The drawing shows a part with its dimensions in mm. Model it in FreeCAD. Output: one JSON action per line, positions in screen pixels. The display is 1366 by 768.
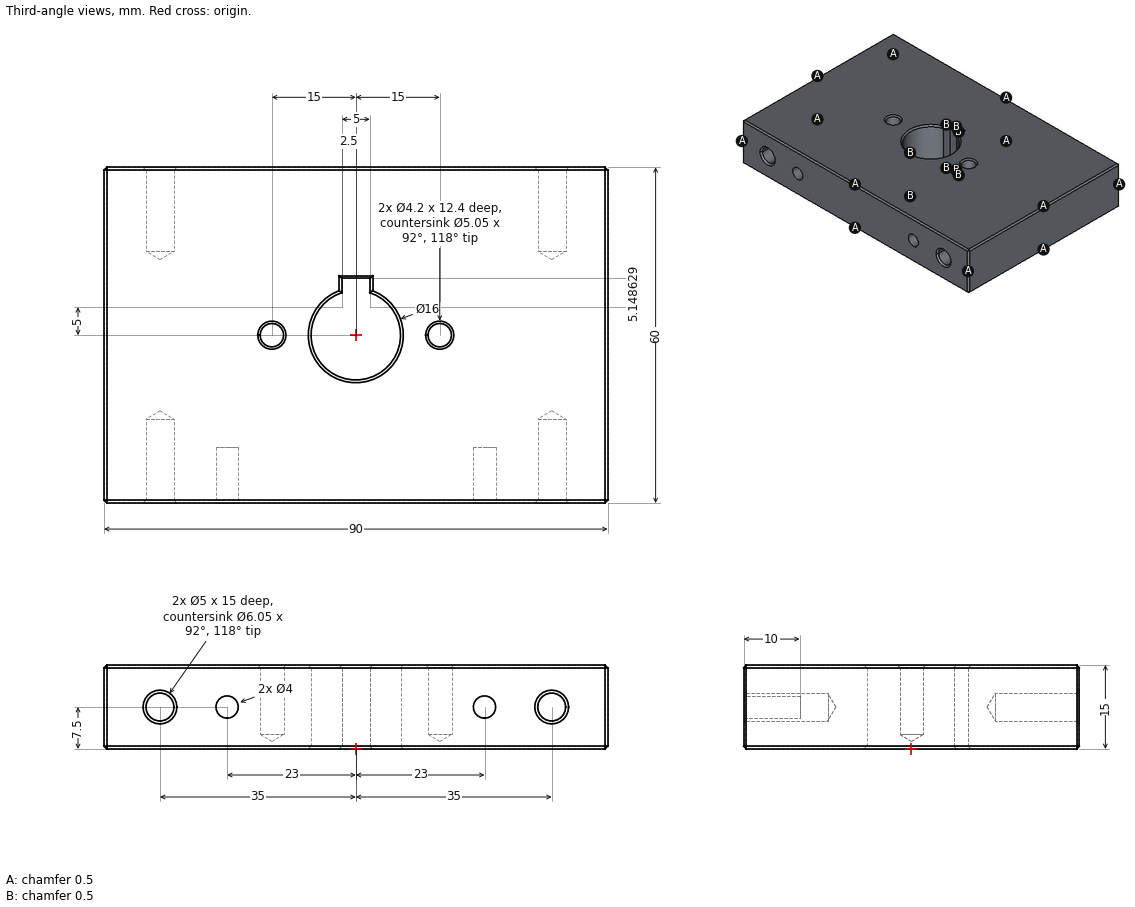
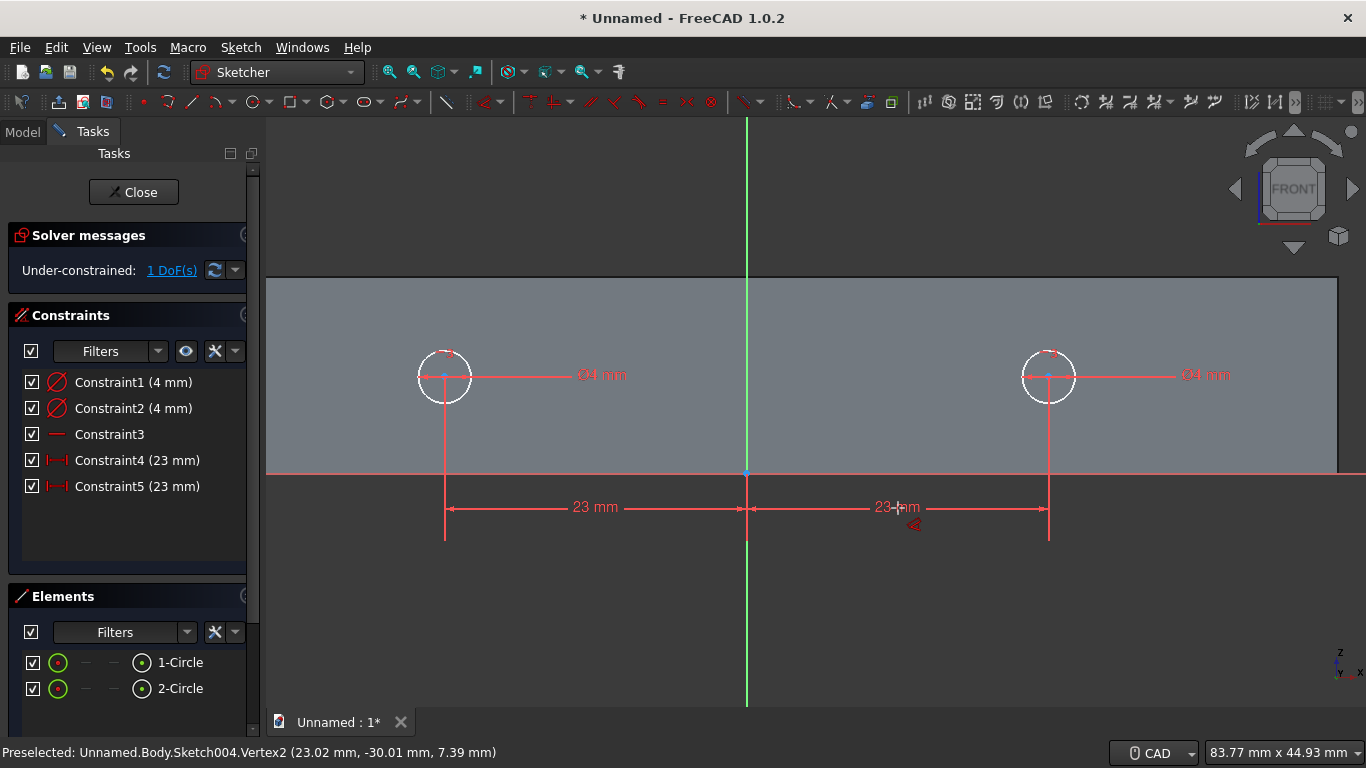
{"action": "left_click", "coordinate": [445, 377]}
{"action": "left_click", "coordinate": [411, 425]}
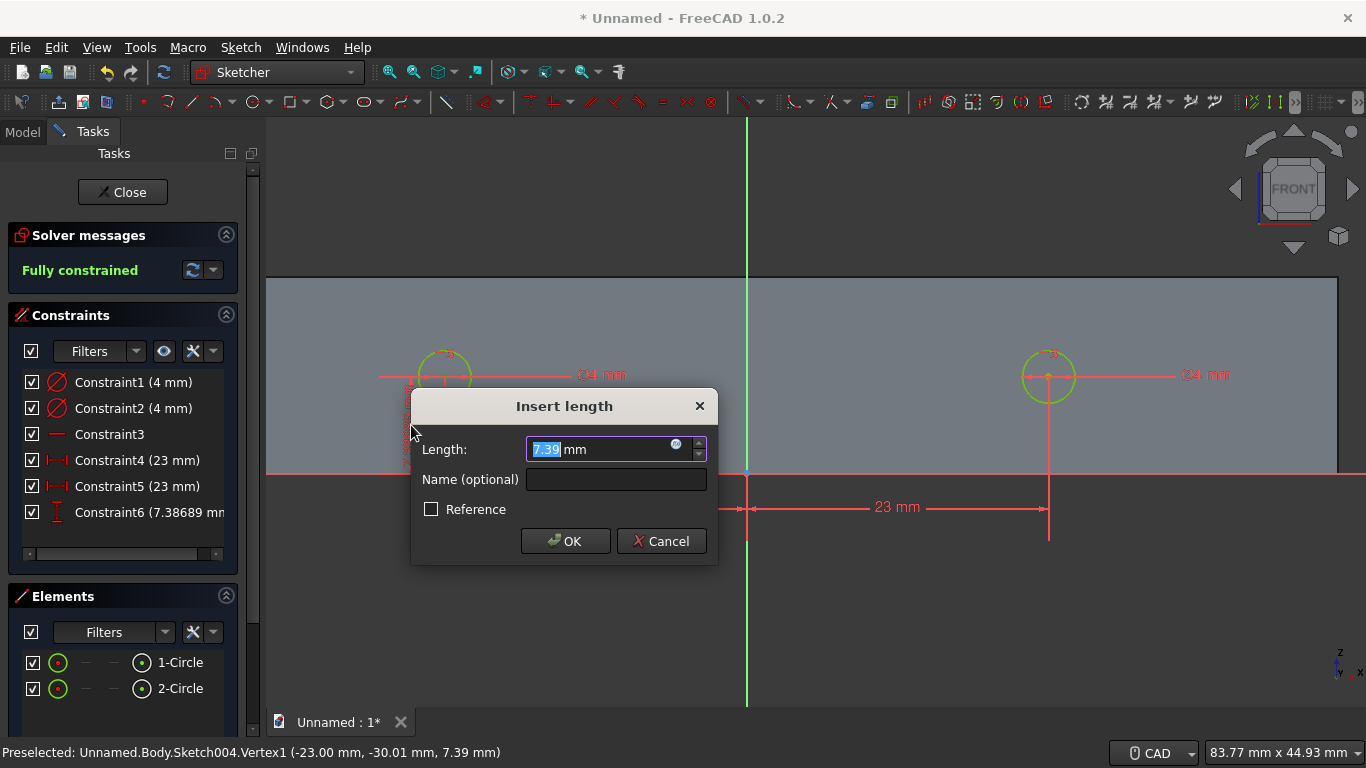
{"action": "type", "text": "7.5"}
{"action": "key", "text": "Return"}
{"action": "key", "text": "Escape"}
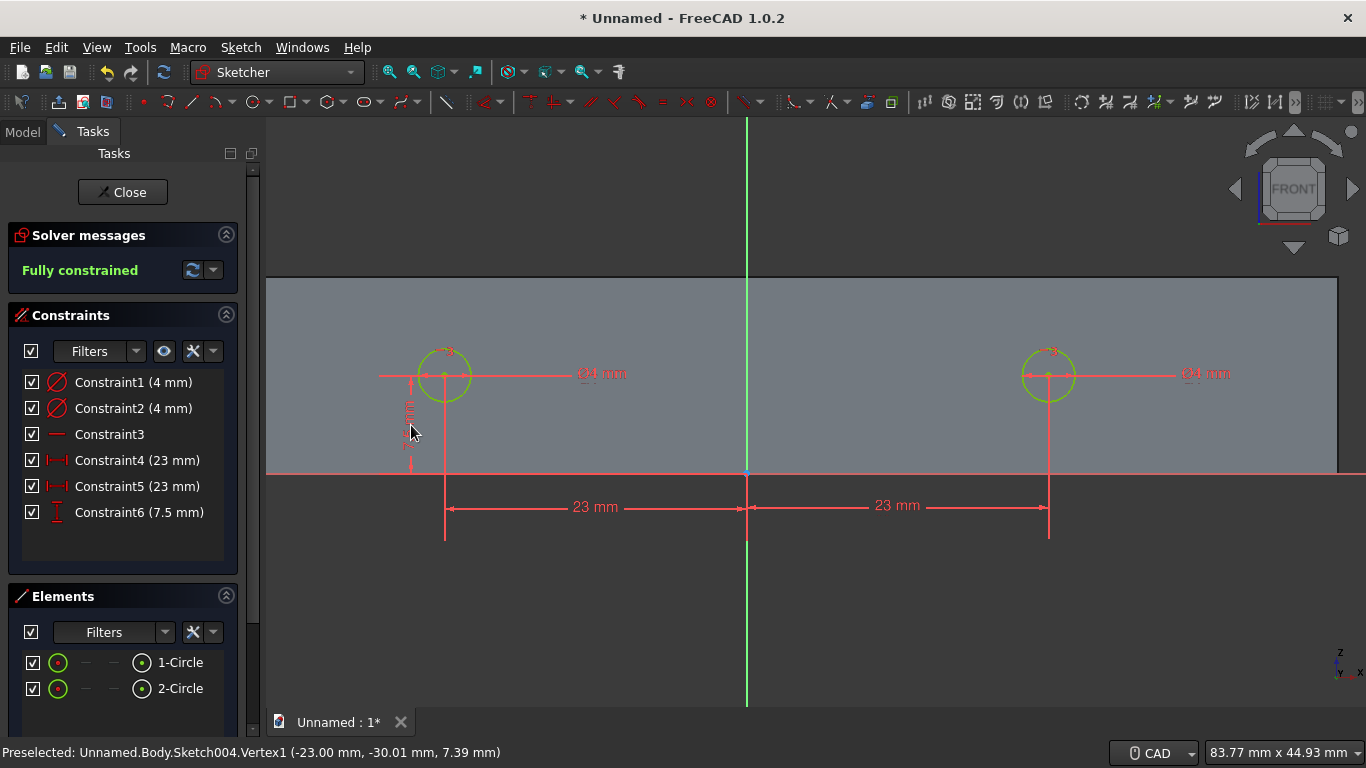
{"action": "left_click", "coordinate": [123, 192]}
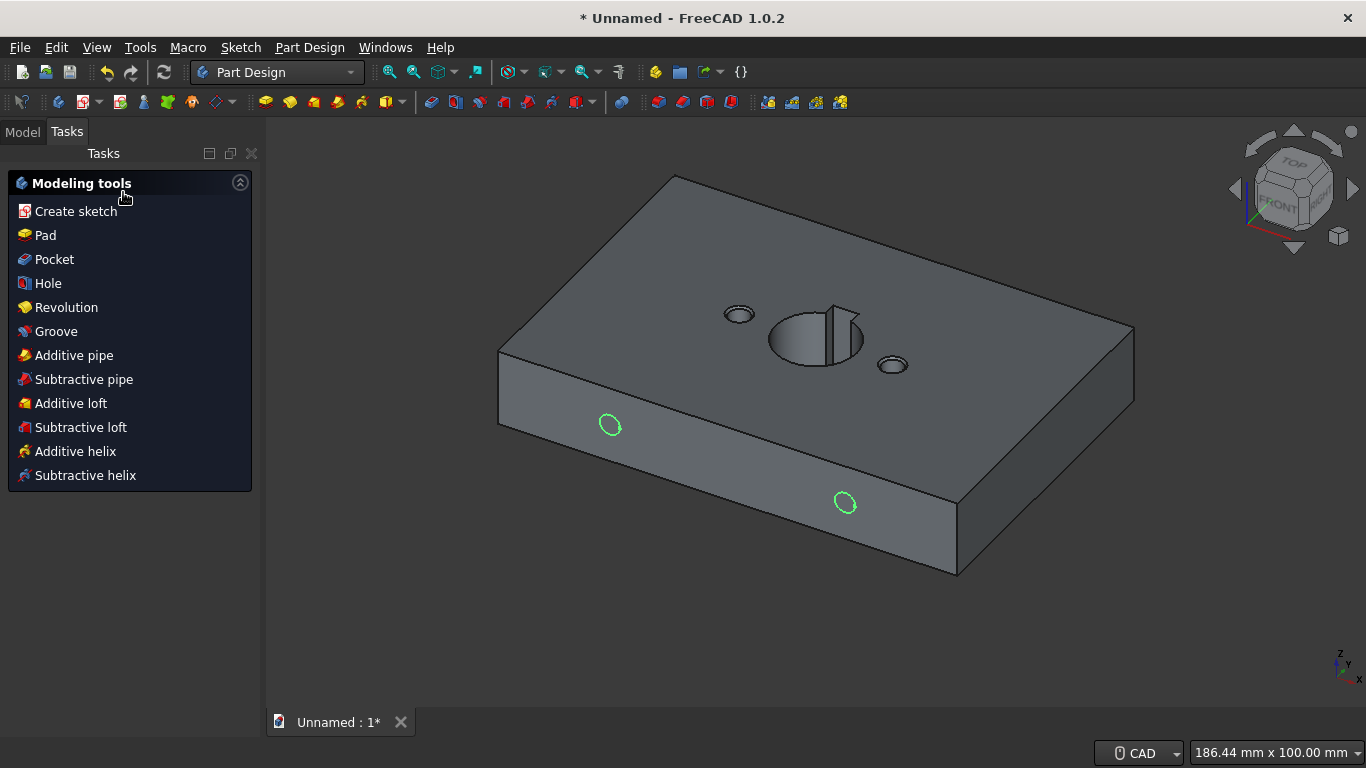
{"action": "left_click", "coordinate": [432, 102]}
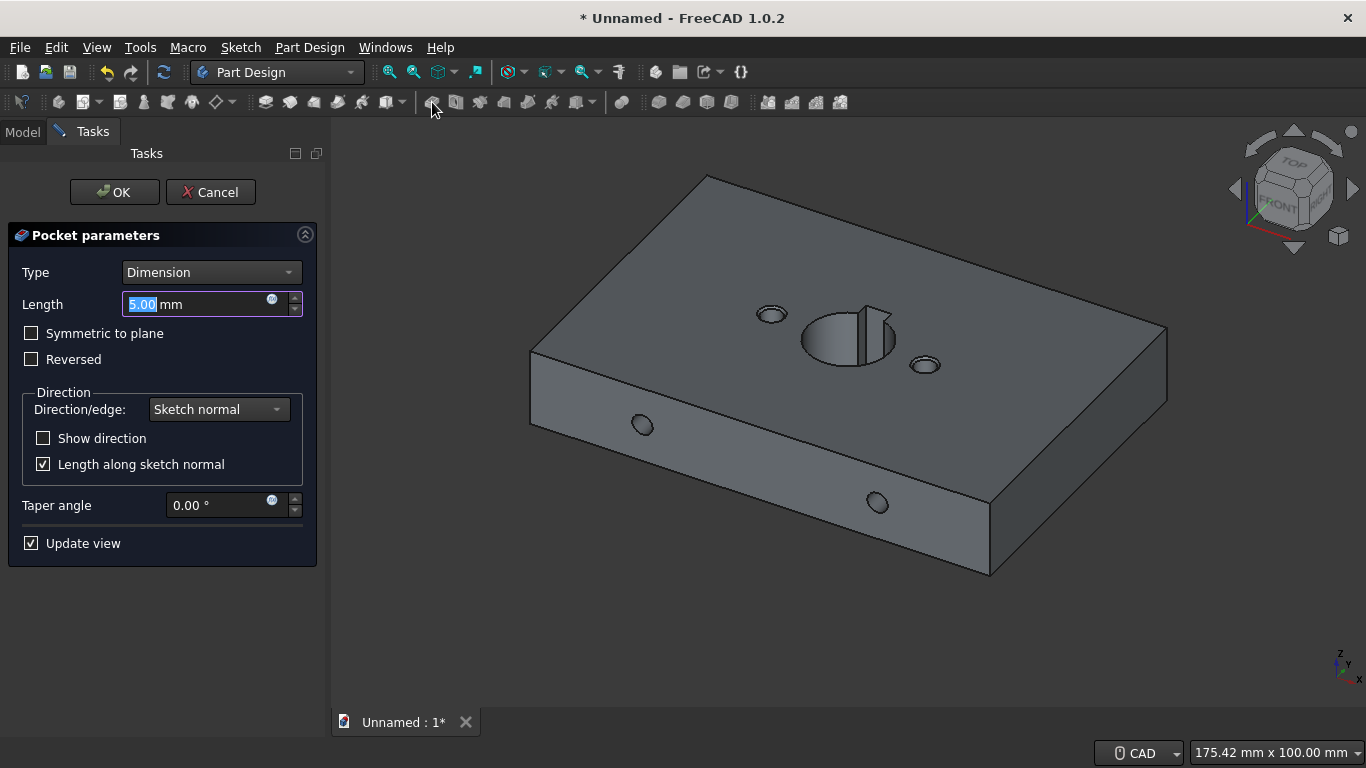
{"action": "type", "text": "10"}
{"action": "key", "text": "Tab"}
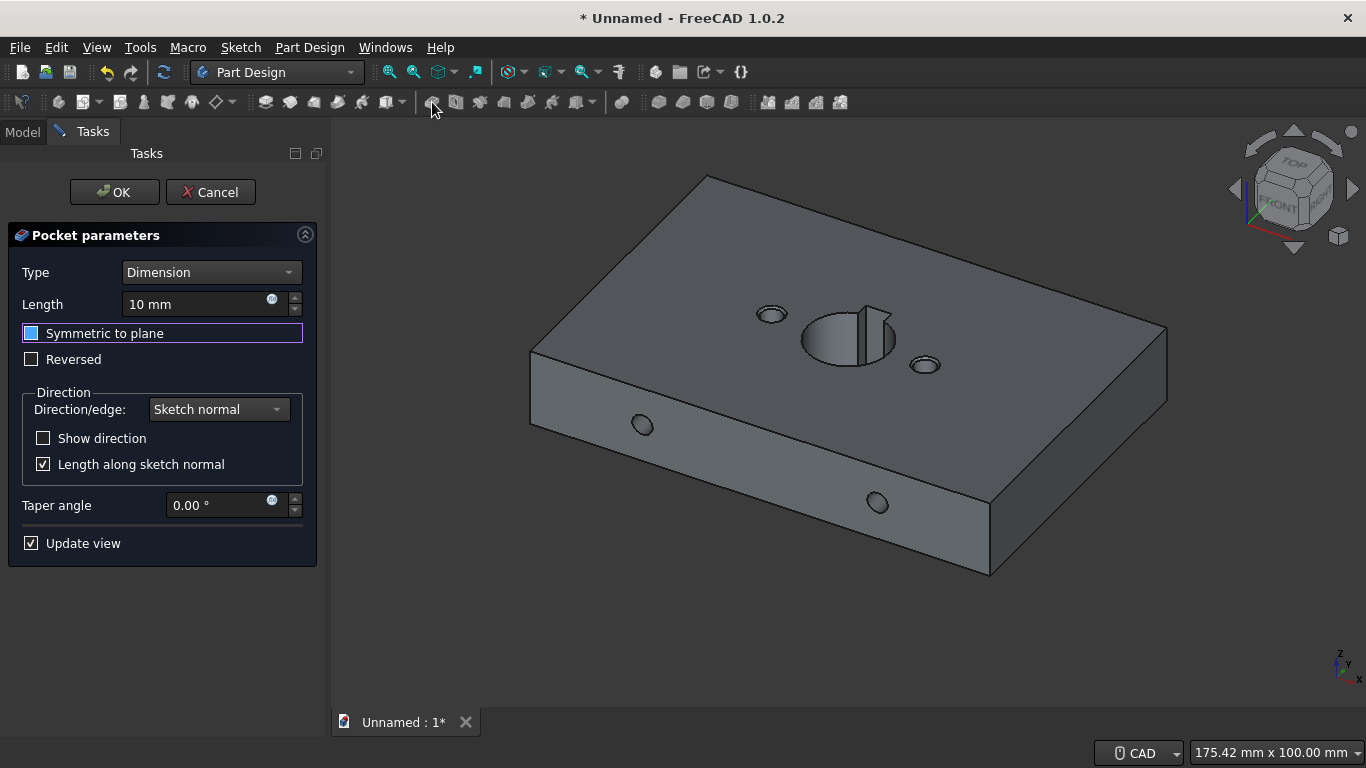
{"action": "left_click", "coordinate": [115, 192]}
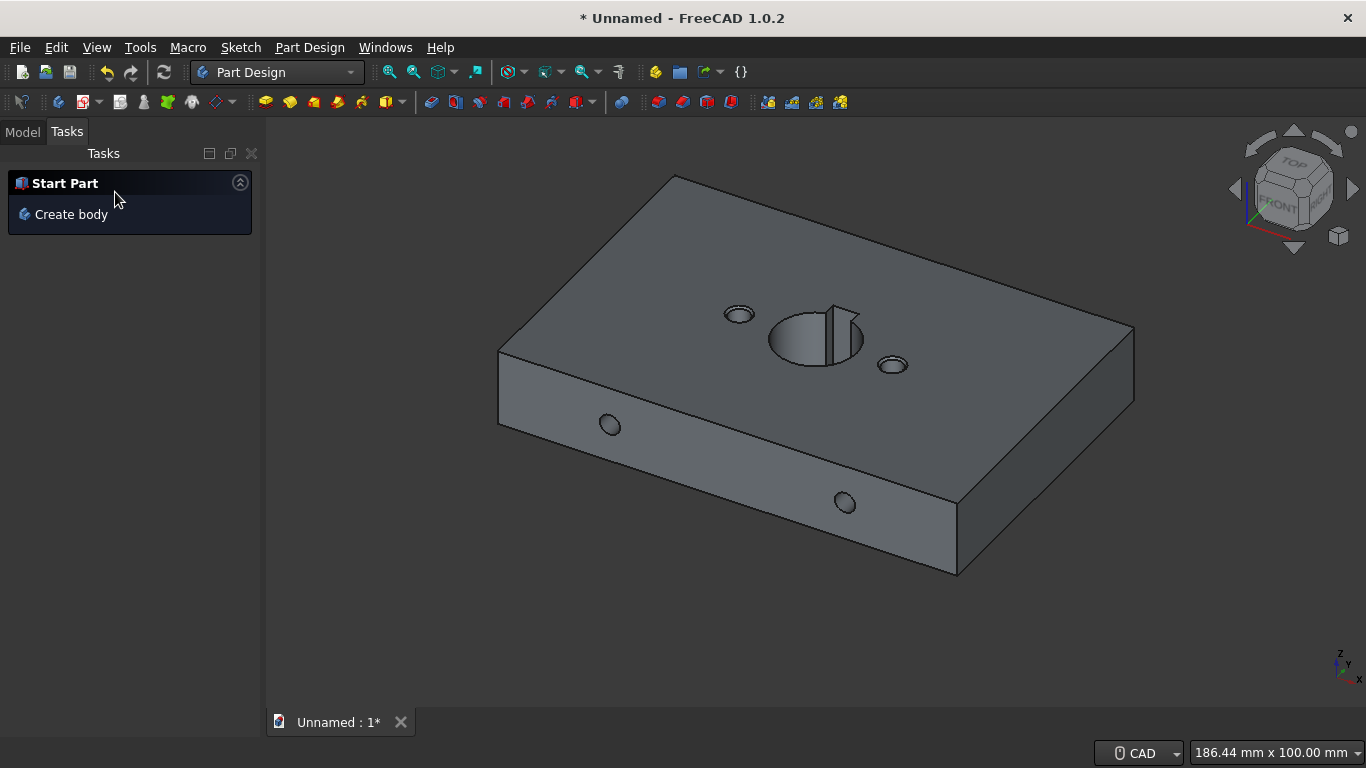
{"action": "key", "text": "4"}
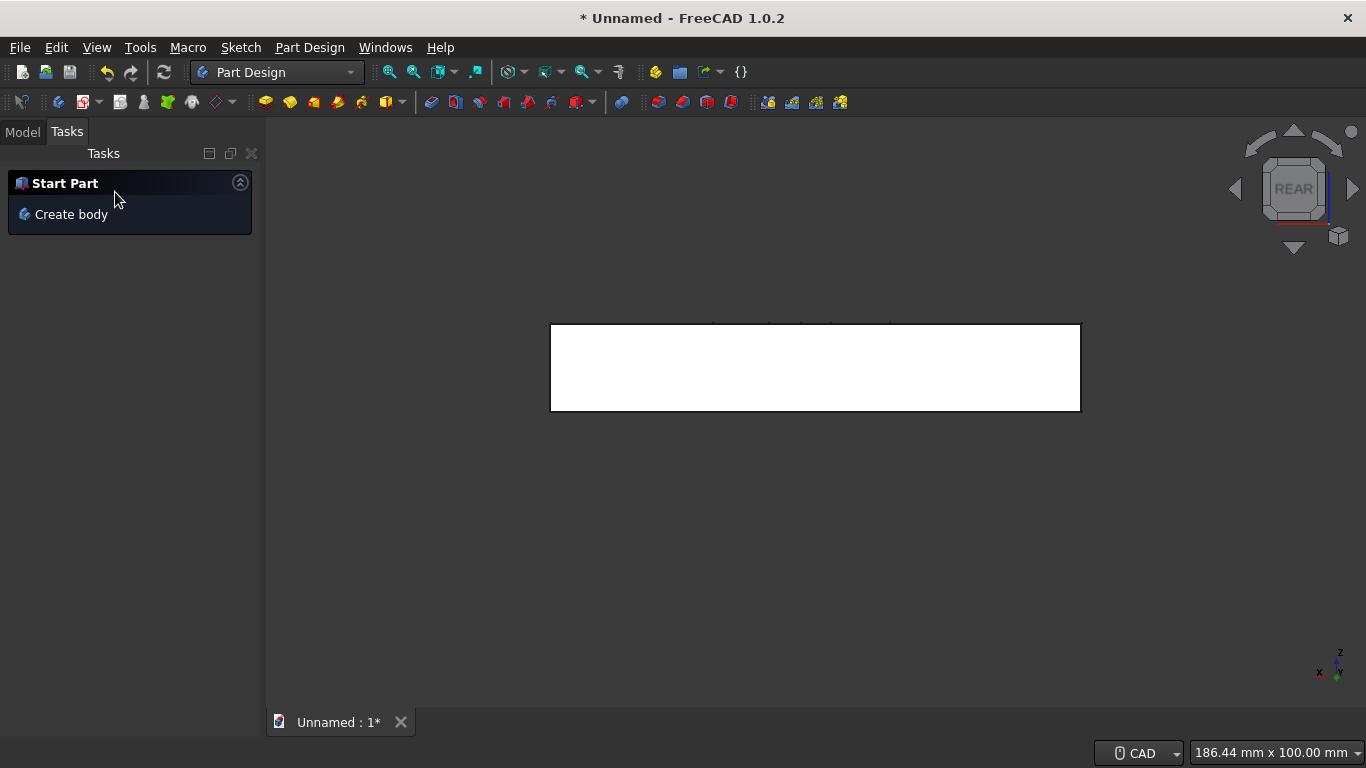
{"action": "left_click", "coordinate": [664, 367]}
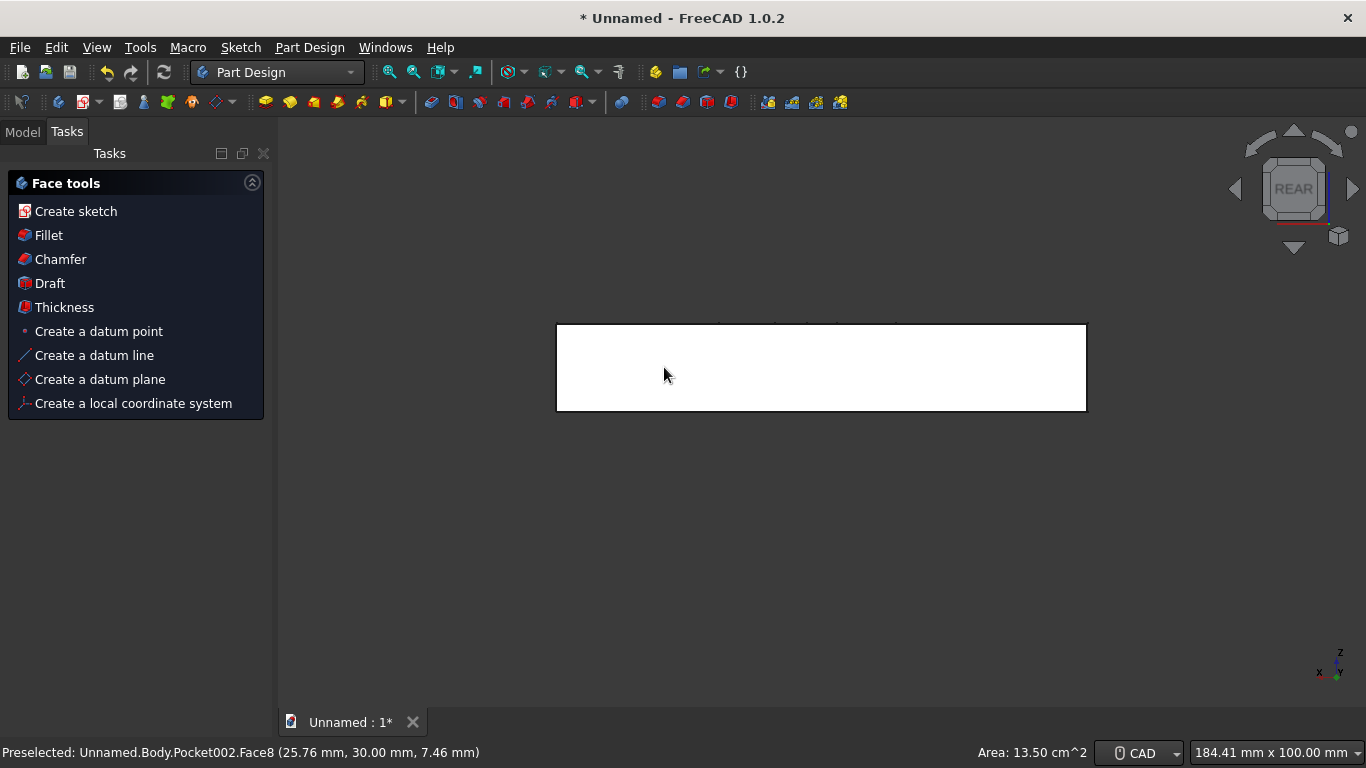
{"action": "left_click", "coordinate": [84, 102]}